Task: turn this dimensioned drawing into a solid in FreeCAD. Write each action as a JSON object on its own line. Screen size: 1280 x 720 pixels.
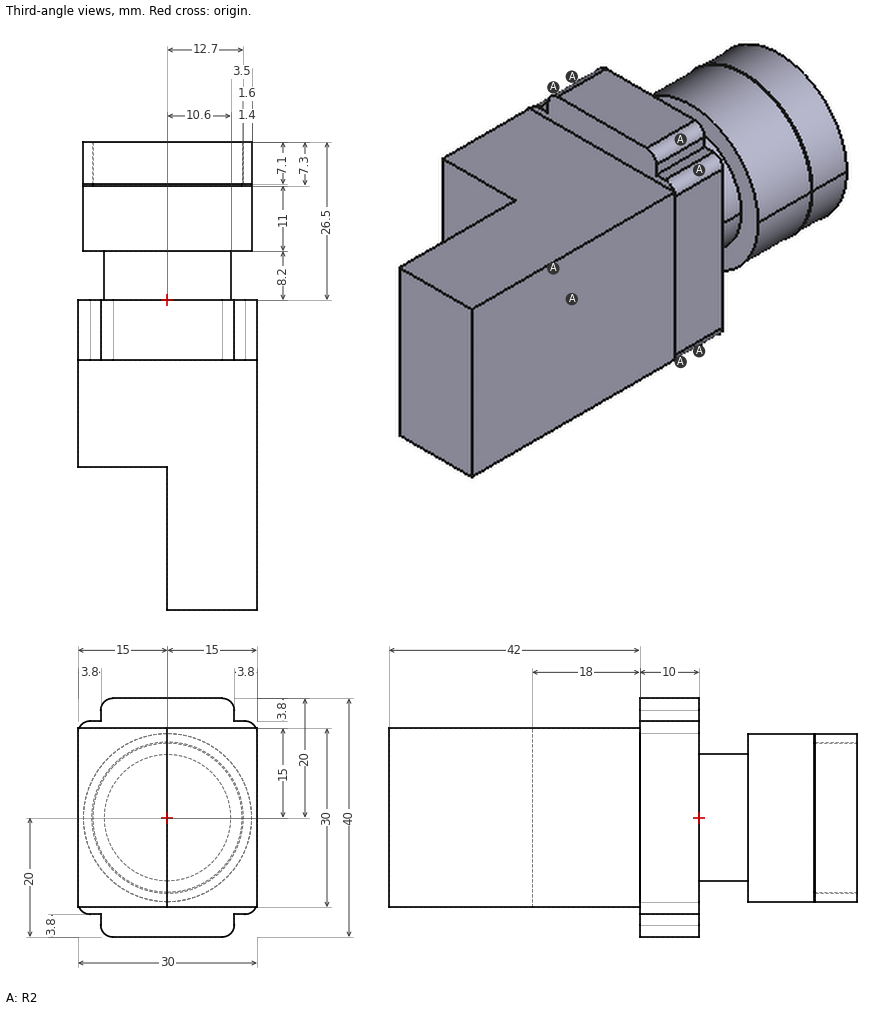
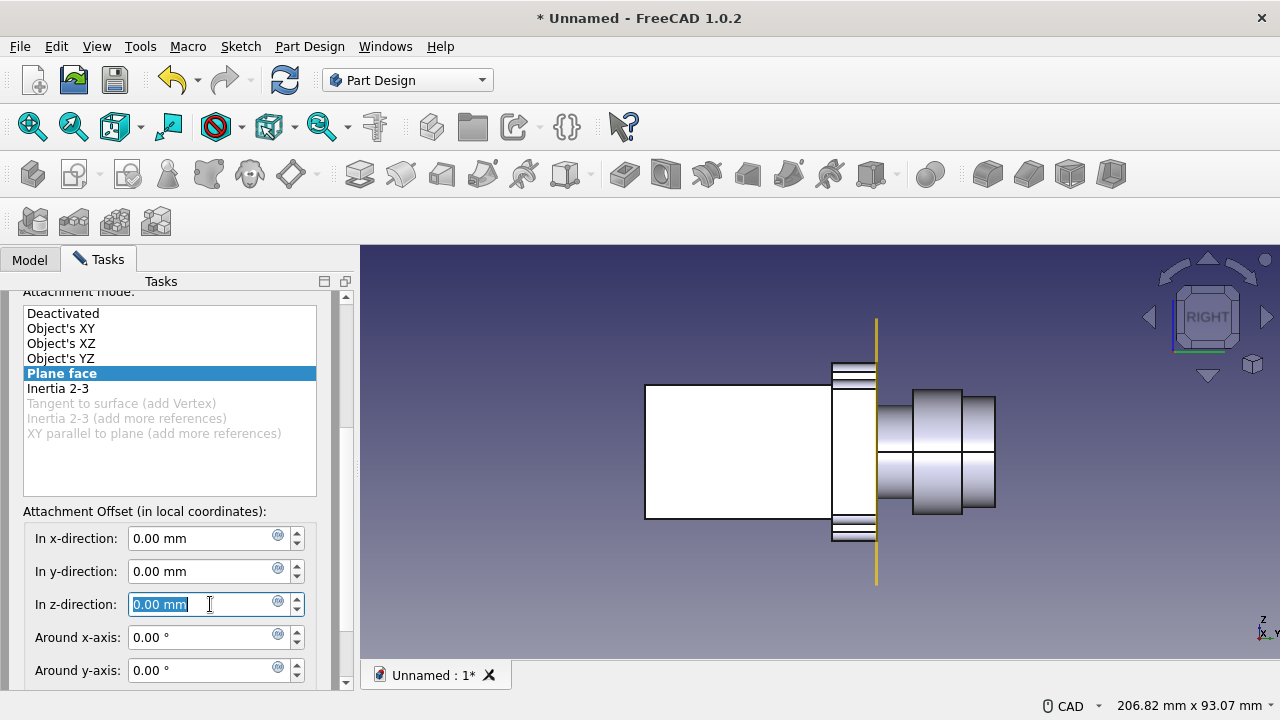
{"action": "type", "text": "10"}
{"action": "key", "text": "Tab"}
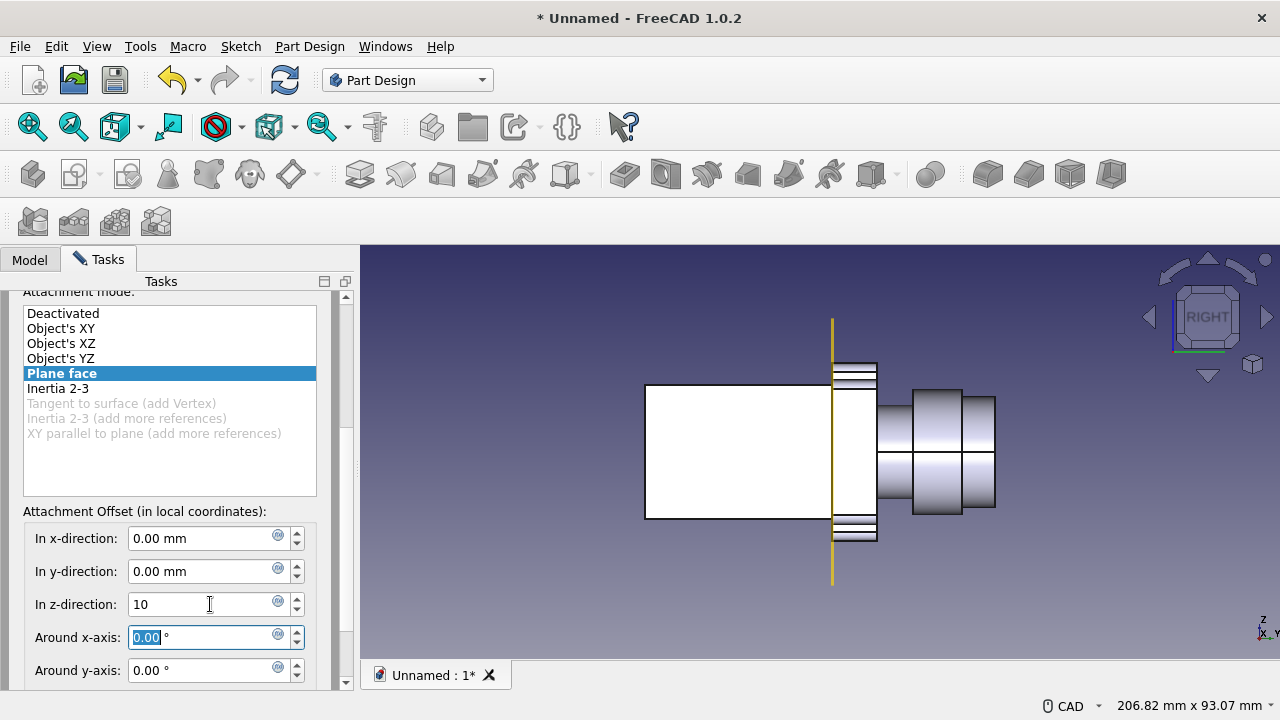
{"action": "scroll", "coordinate": [346, 490], "scroll_direction": "up", "scroll_amount": 5}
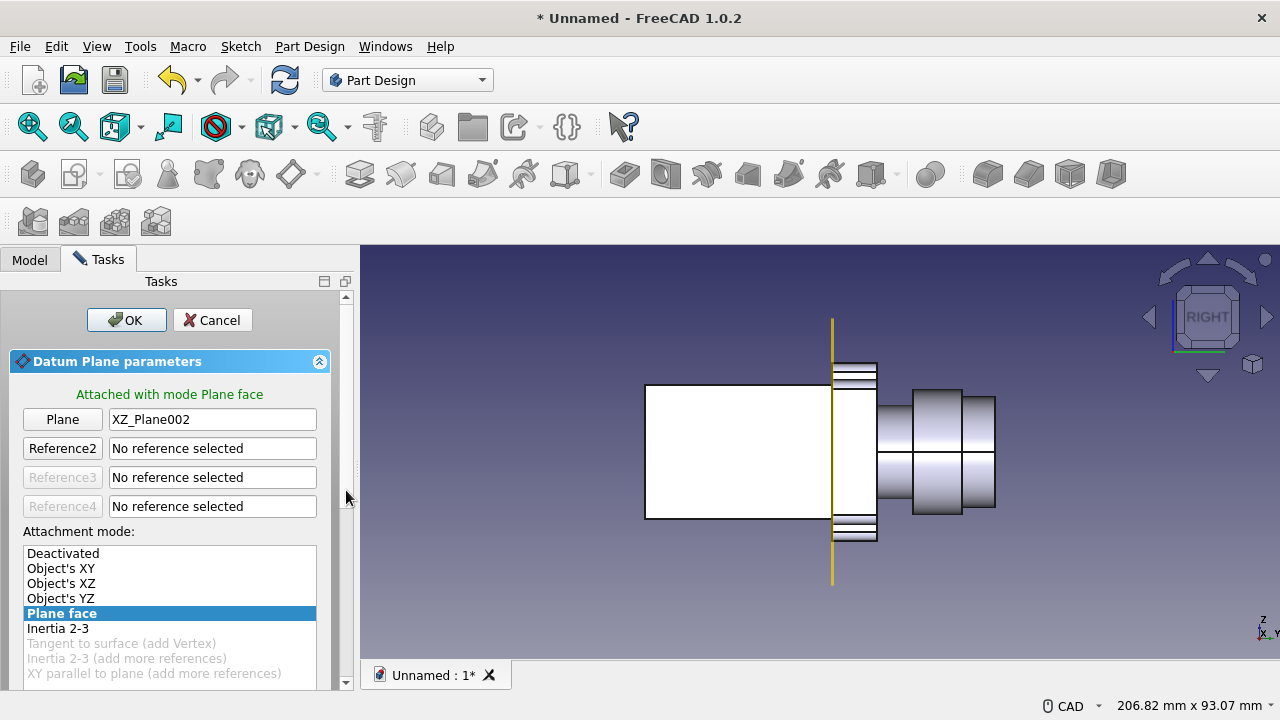
{"action": "left_click", "coordinate": [127, 320]}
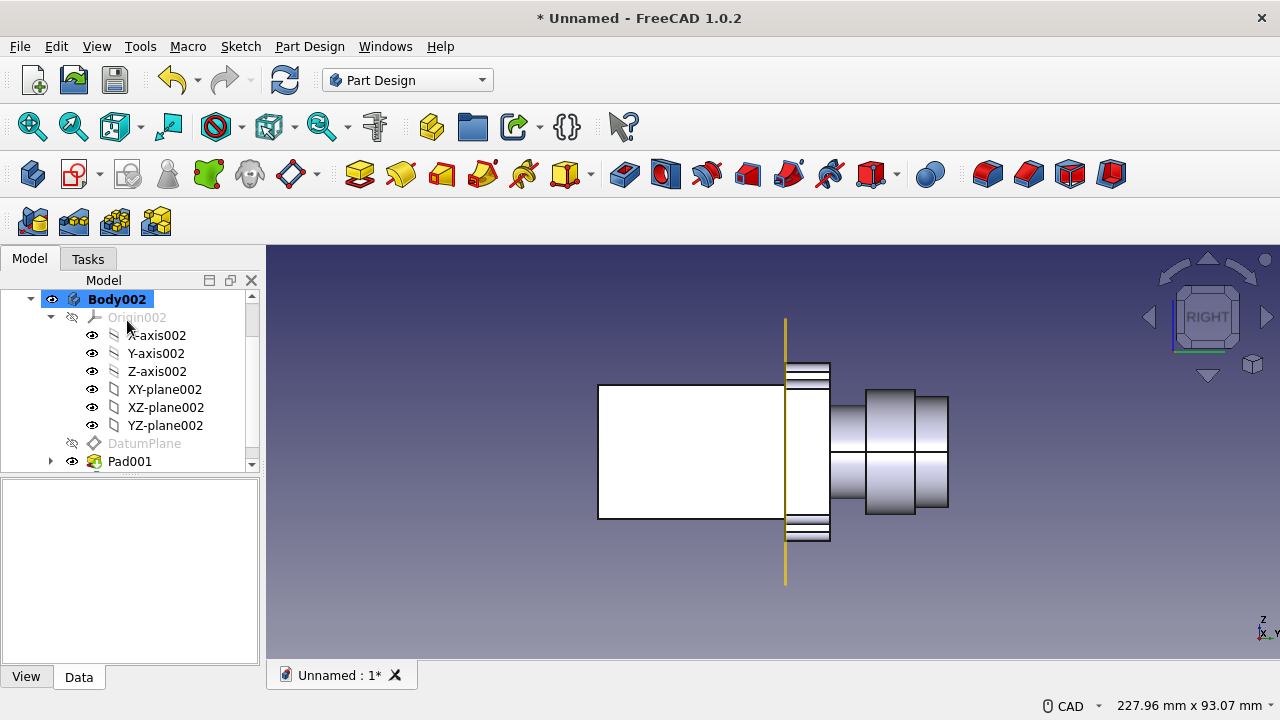
{"action": "scroll", "coordinate": [121, 385], "scroll_direction": "down", "scroll_amount": 3}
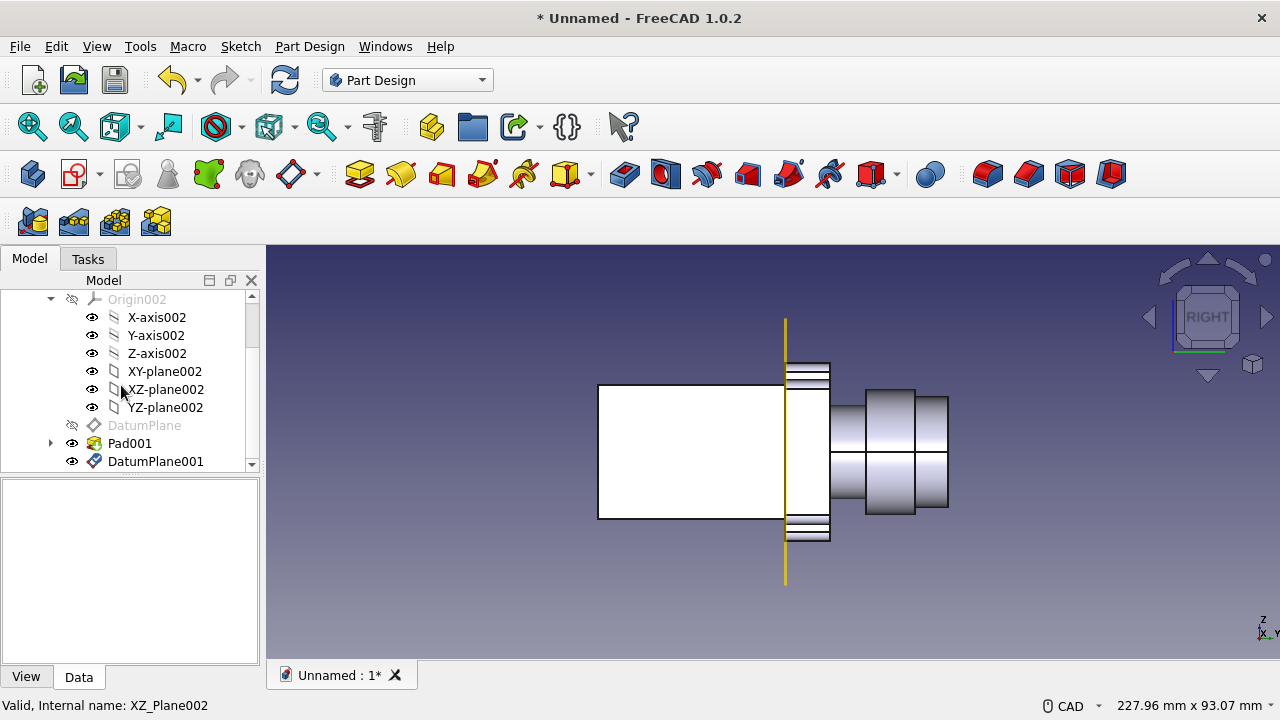
{"action": "left_click", "coordinate": [117, 461]}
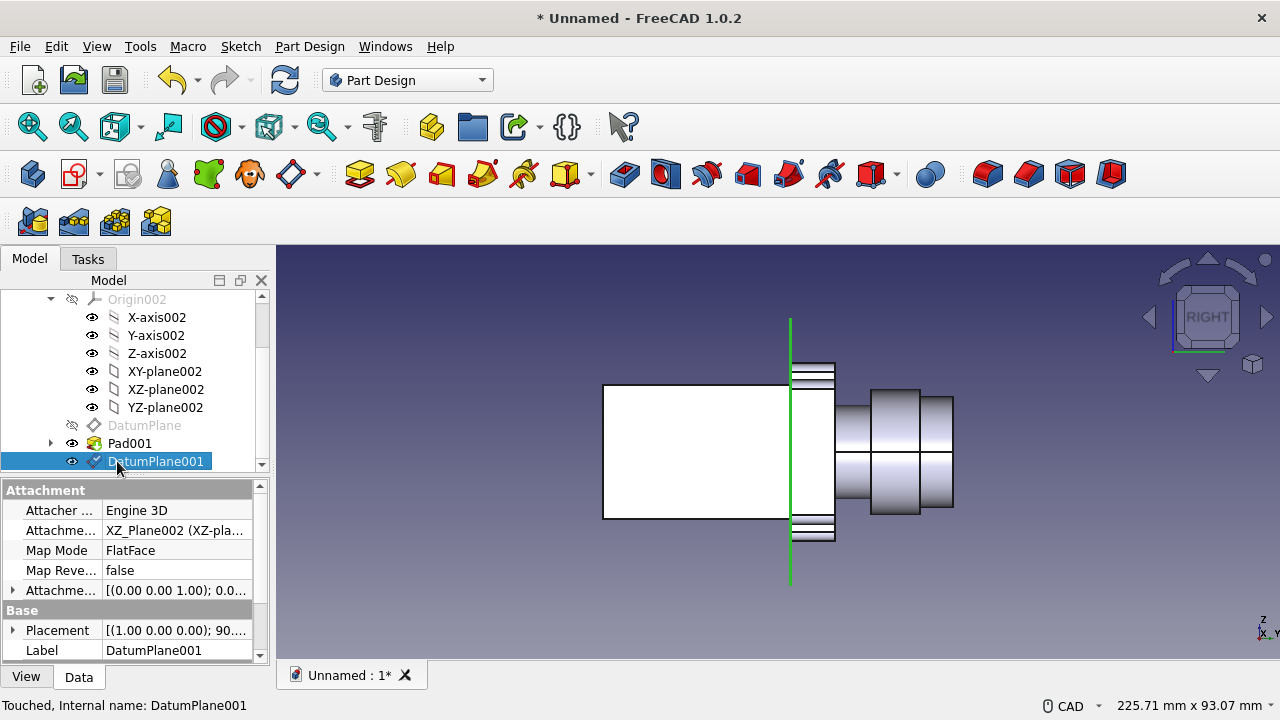
{"action": "left_click", "coordinate": [74, 174]}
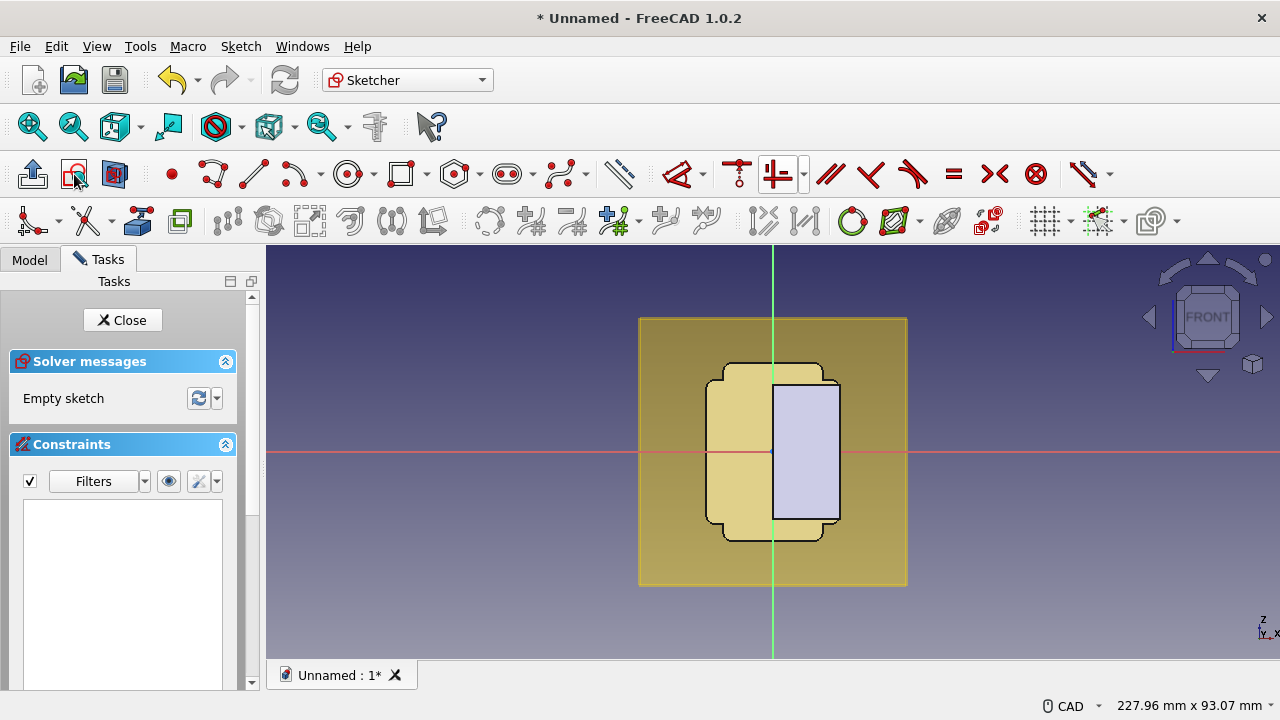
{"action": "key", "text": "q s"}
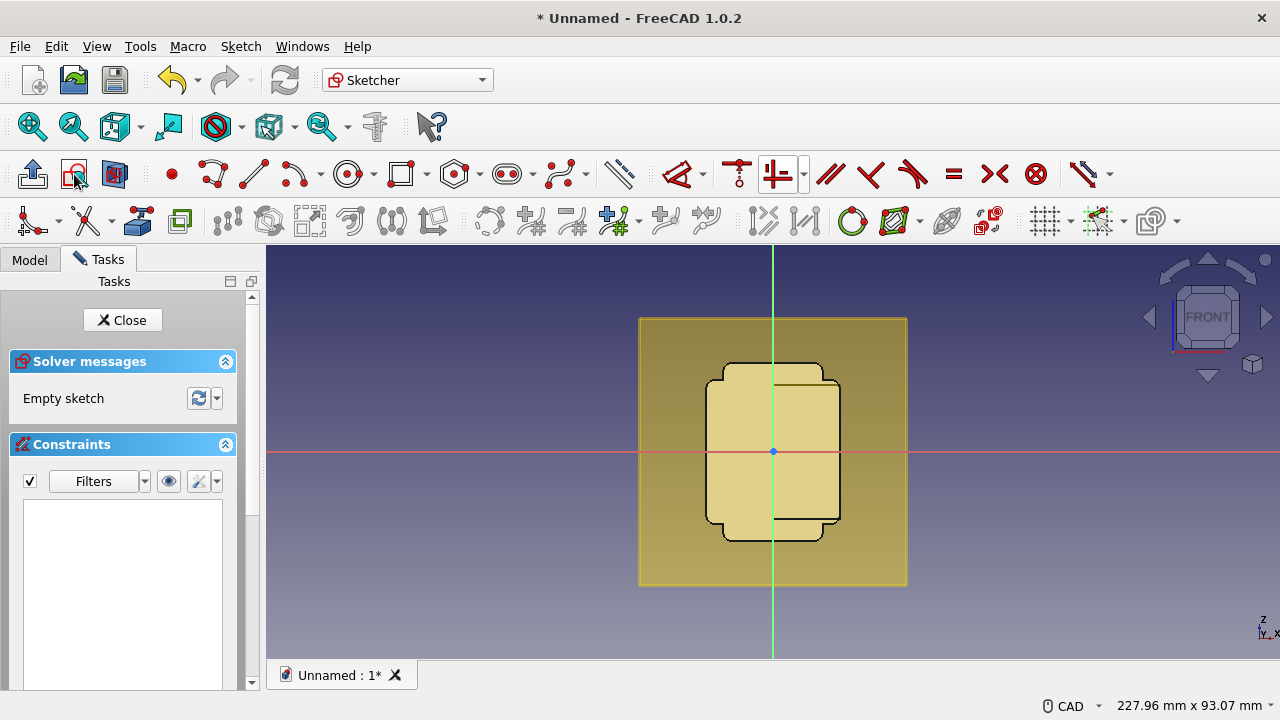
{"action": "scroll", "coordinate": [782, 452], "scroll_direction": "up", "scroll_amount": 3}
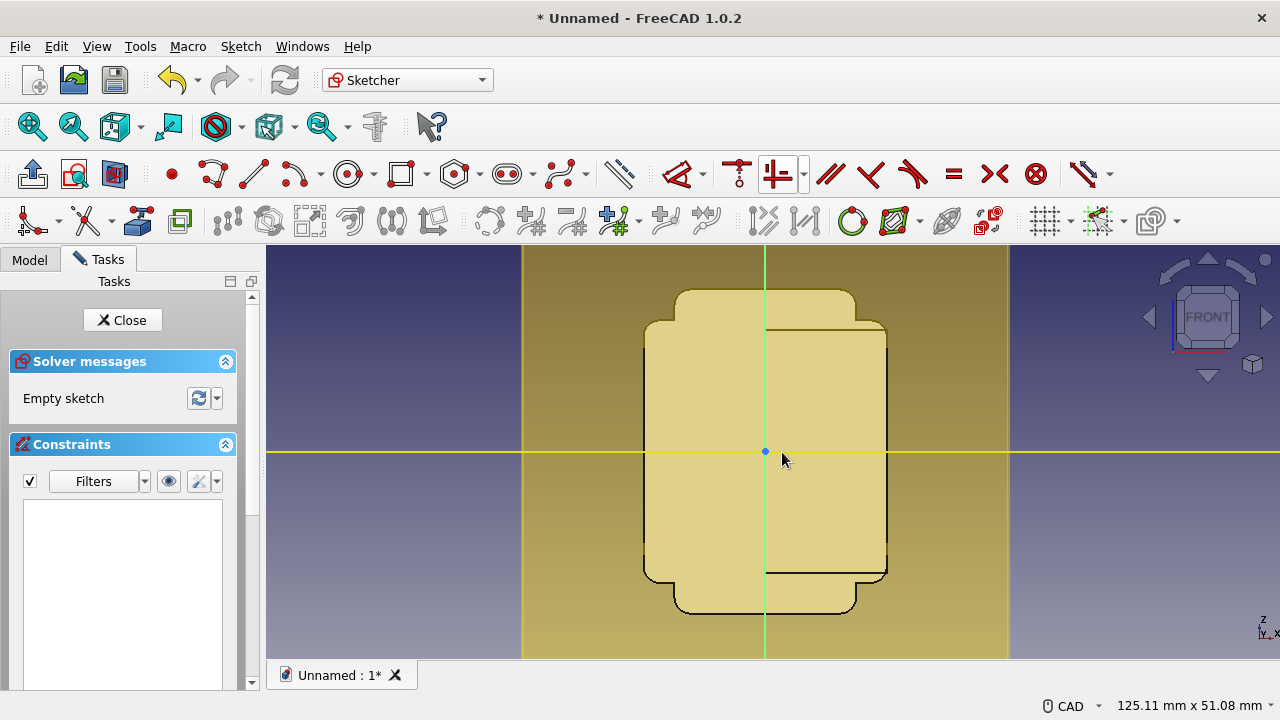
{"action": "left_click", "coordinate": [400, 174]}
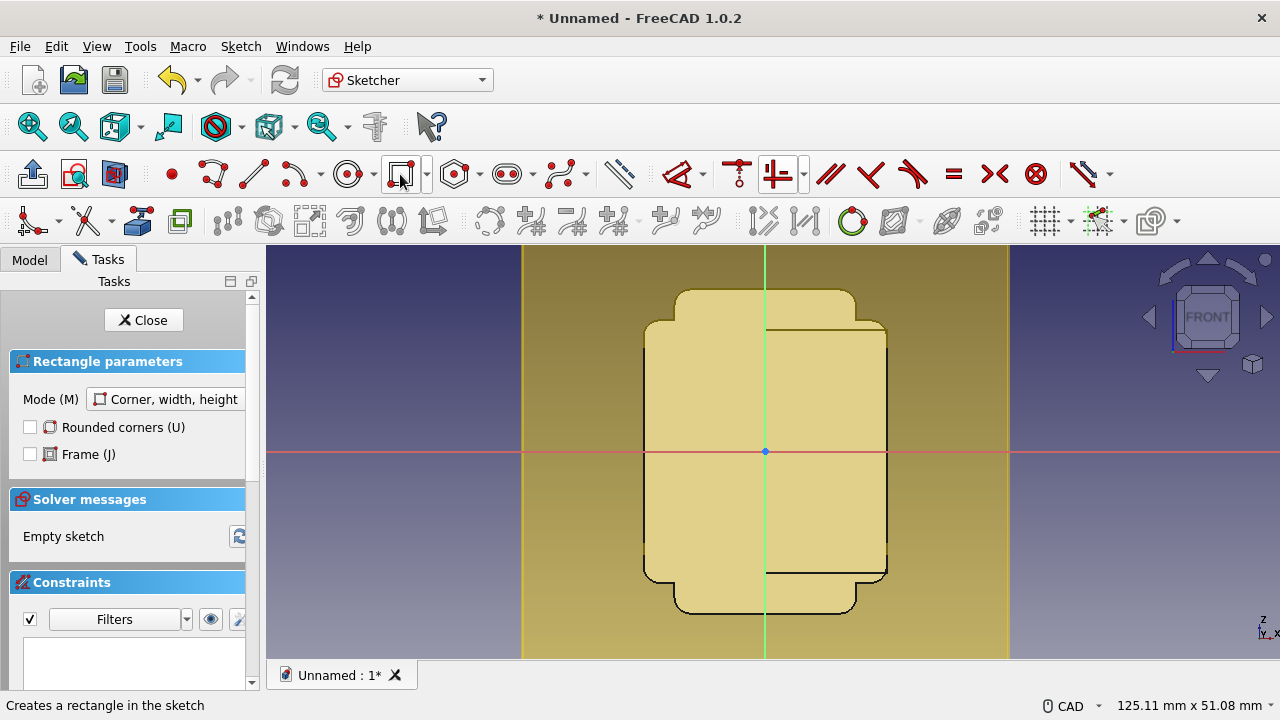
{"action": "left_click", "coordinate": [644, 330]}
{"action": "left_click", "coordinate": [765, 573]}
{"action": "key", "text": "Escape"}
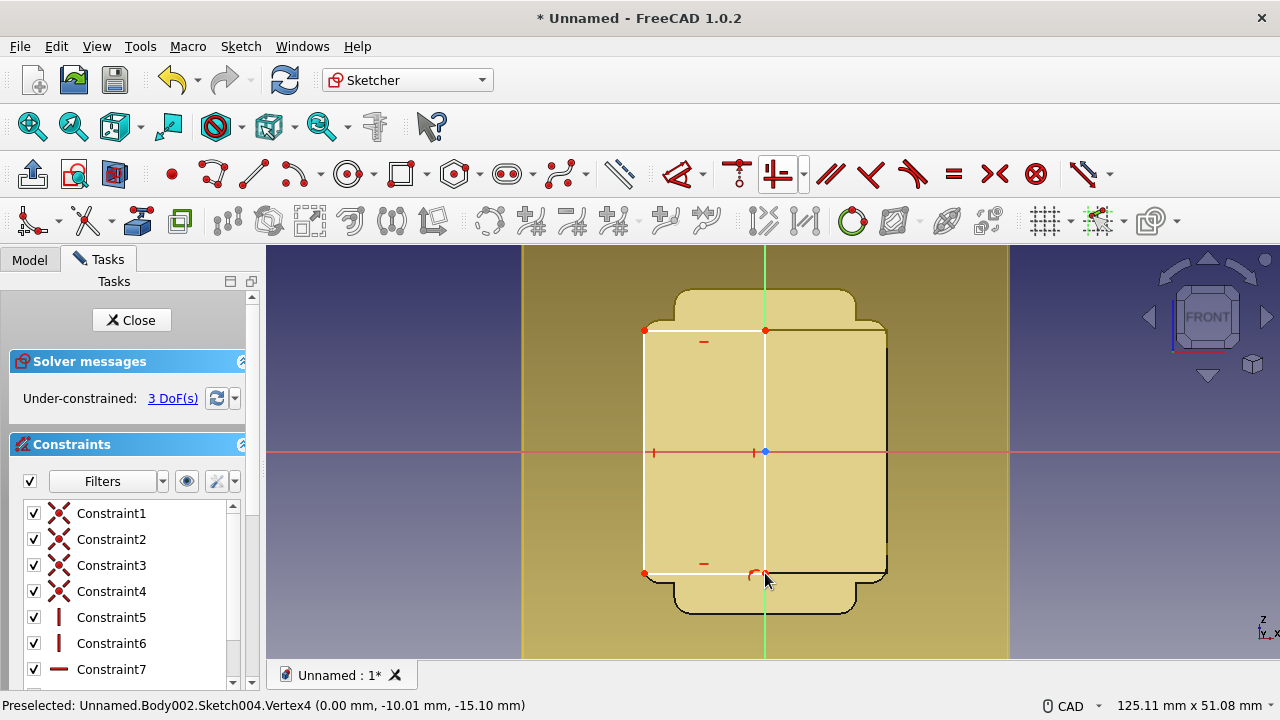
{"action": "left_click", "coordinate": [676, 174]}